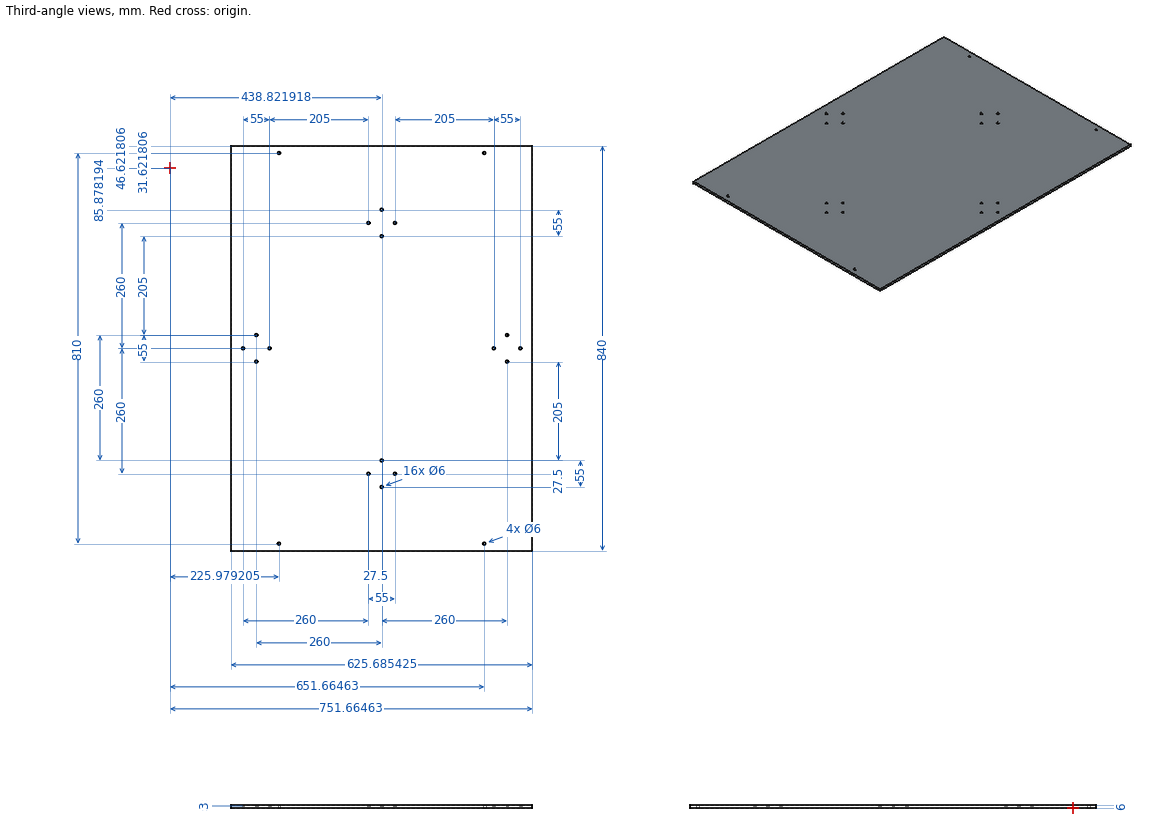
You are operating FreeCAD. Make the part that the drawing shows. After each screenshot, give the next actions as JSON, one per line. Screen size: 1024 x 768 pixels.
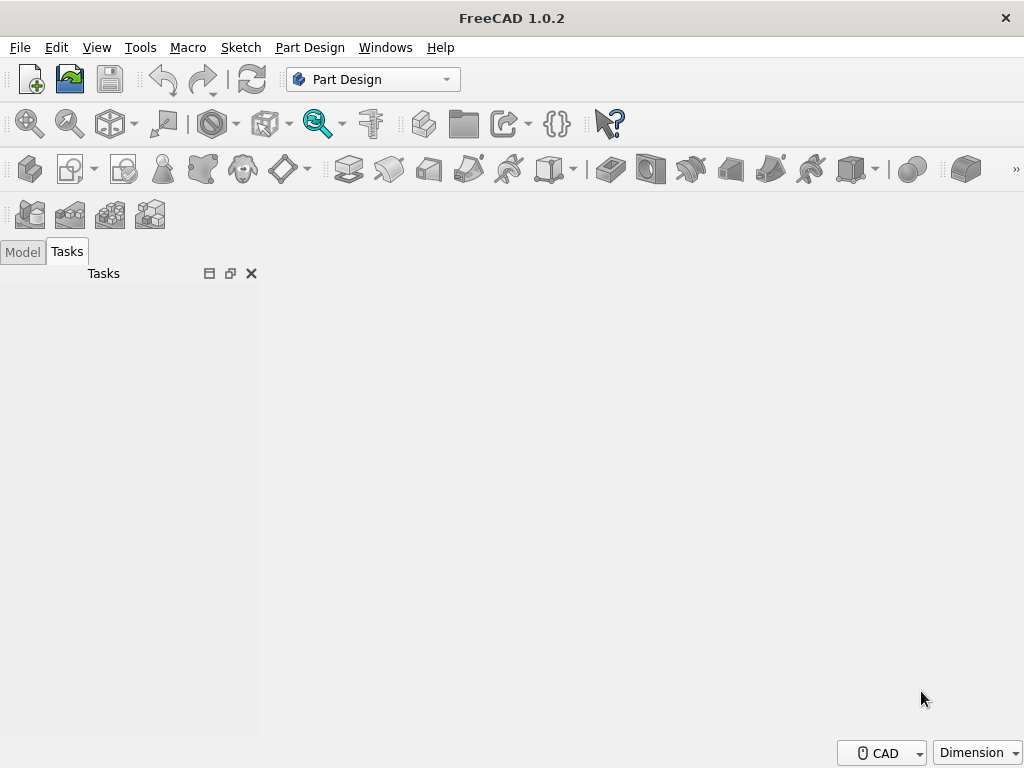
{"action": "left_click", "coordinate": [30, 80]}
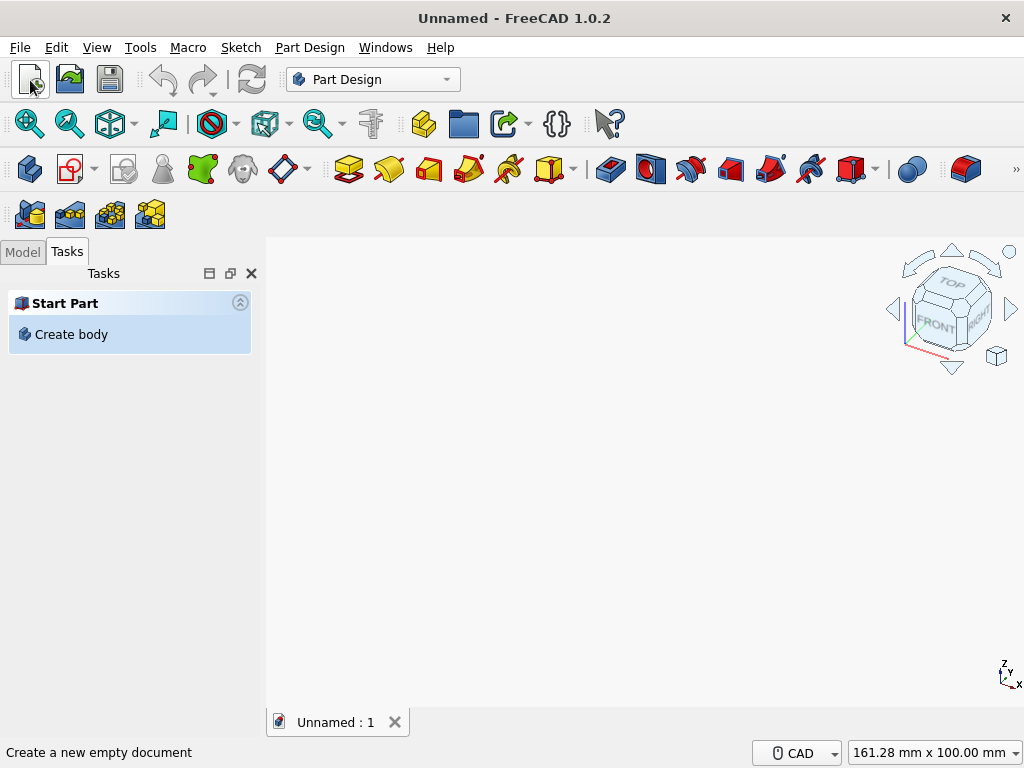
{"action": "left_click", "coordinate": [70, 170]}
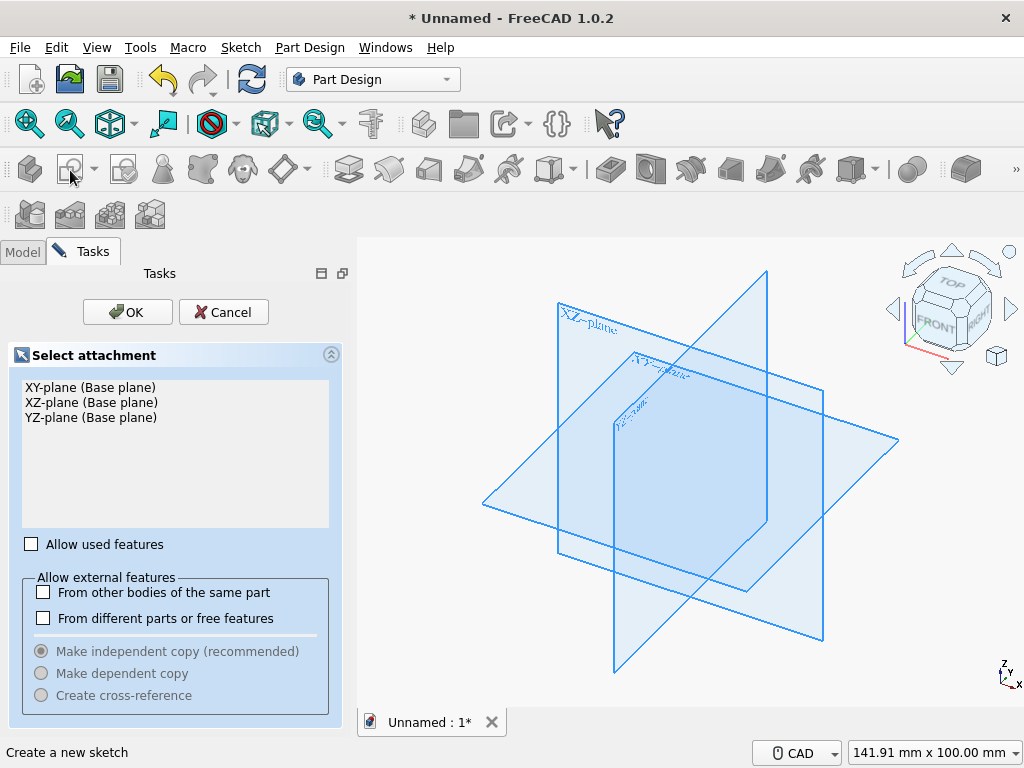
{"action": "left_click", "coordinate": [82, 388]}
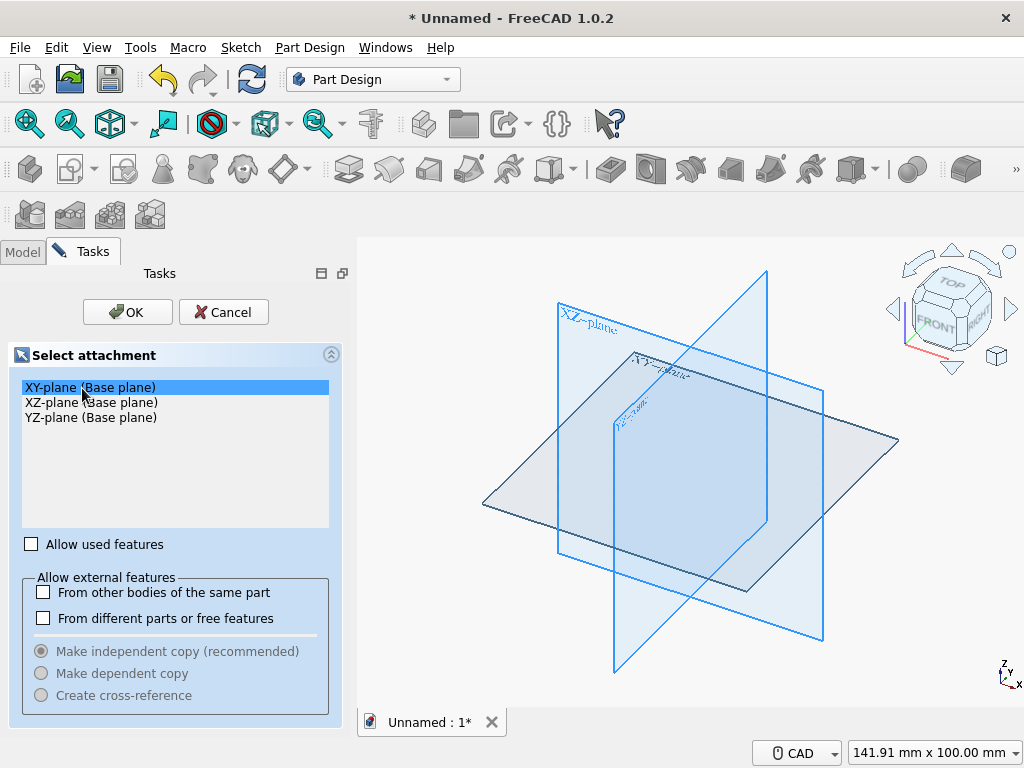
{"action": "left_click", "coordinate": [128, 312]}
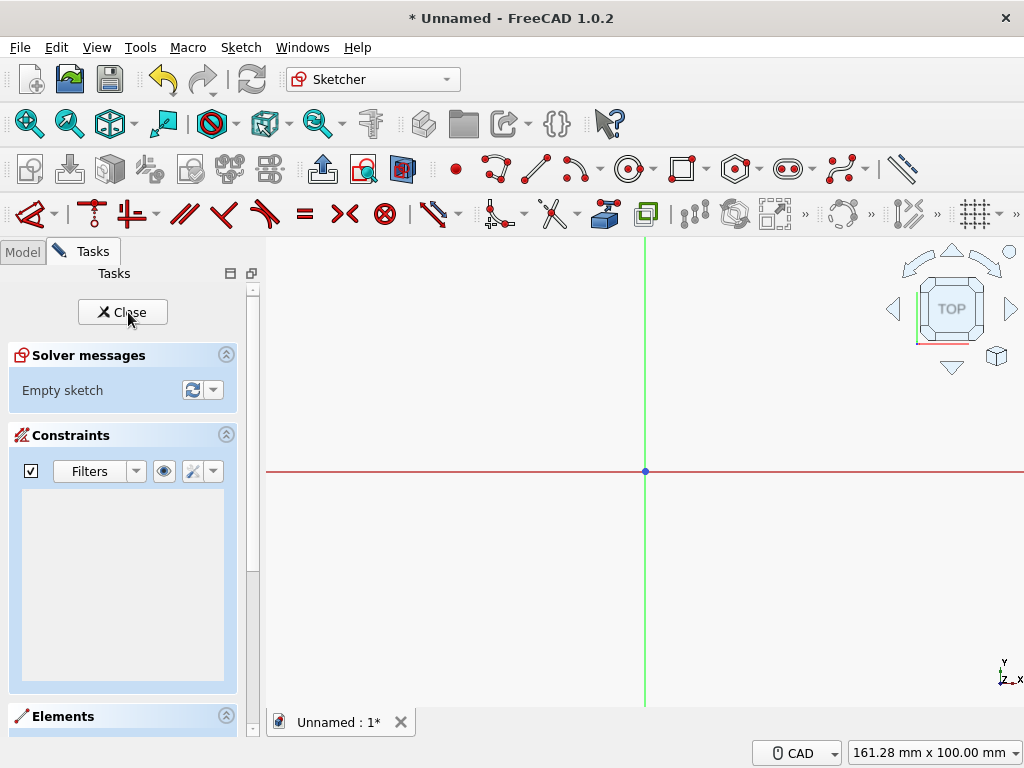
{"action": "scroll", "coordinate": [429, 331], "scroll_direction": "down", "scroll_amount": 13}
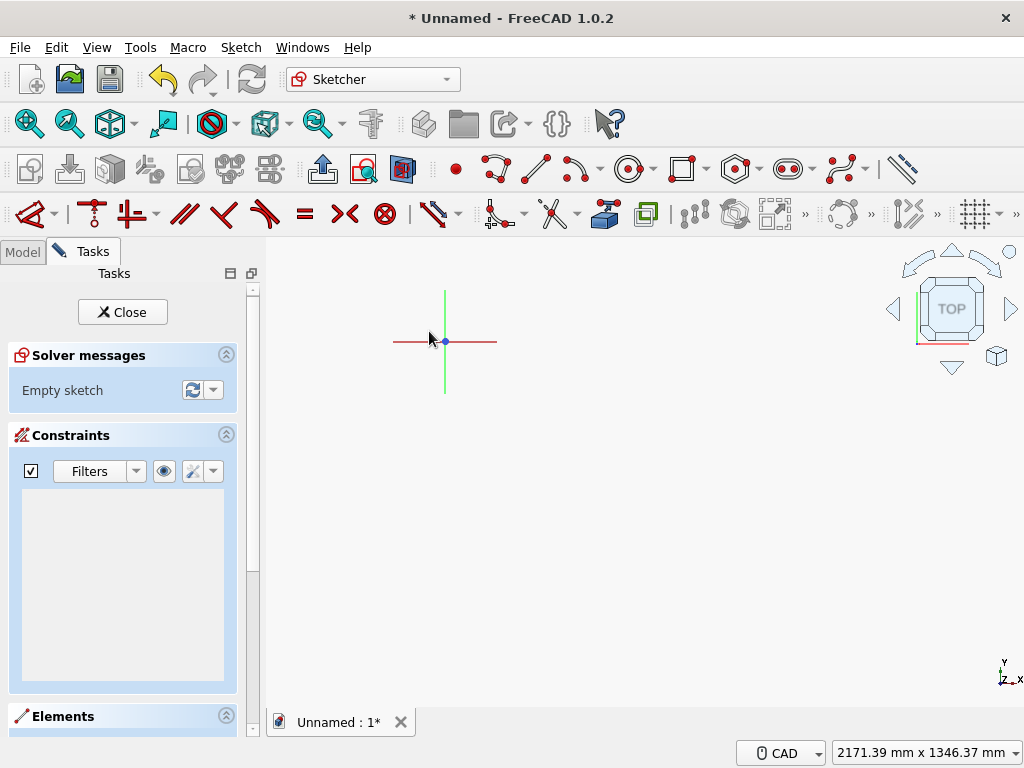
{"action": "left_click", "coordinate": [682, 170]}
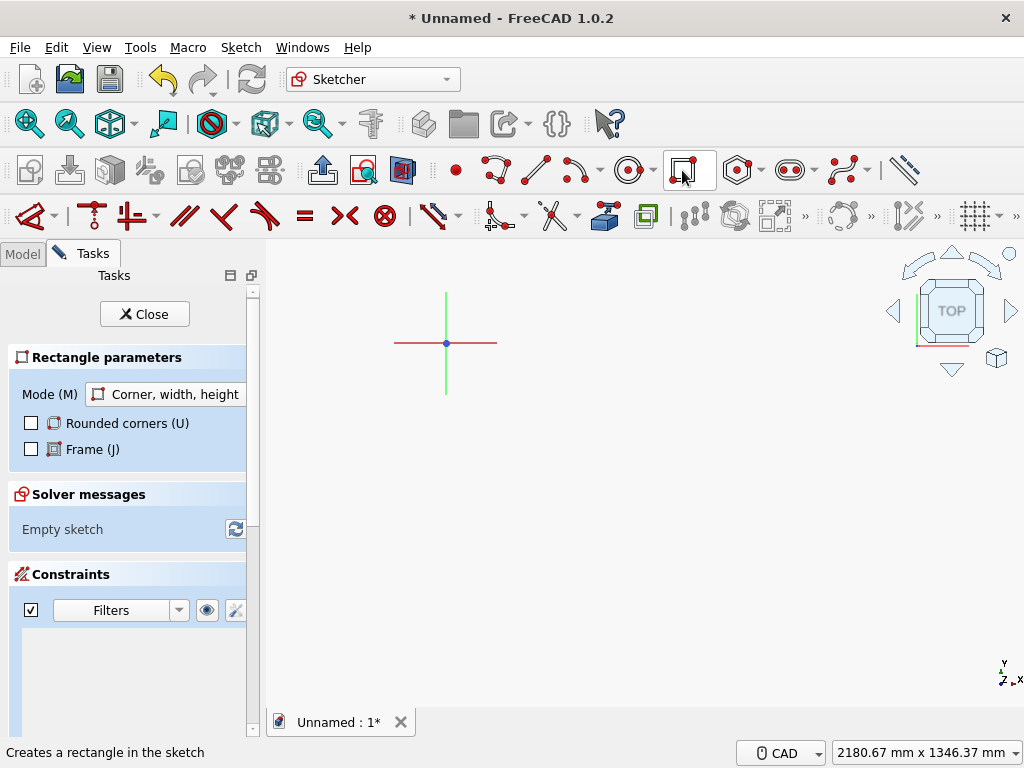
{"action": "left_click", "coordinate": [490, 327]}
{"action": "mouse_move", "coordinate": [707, 619]}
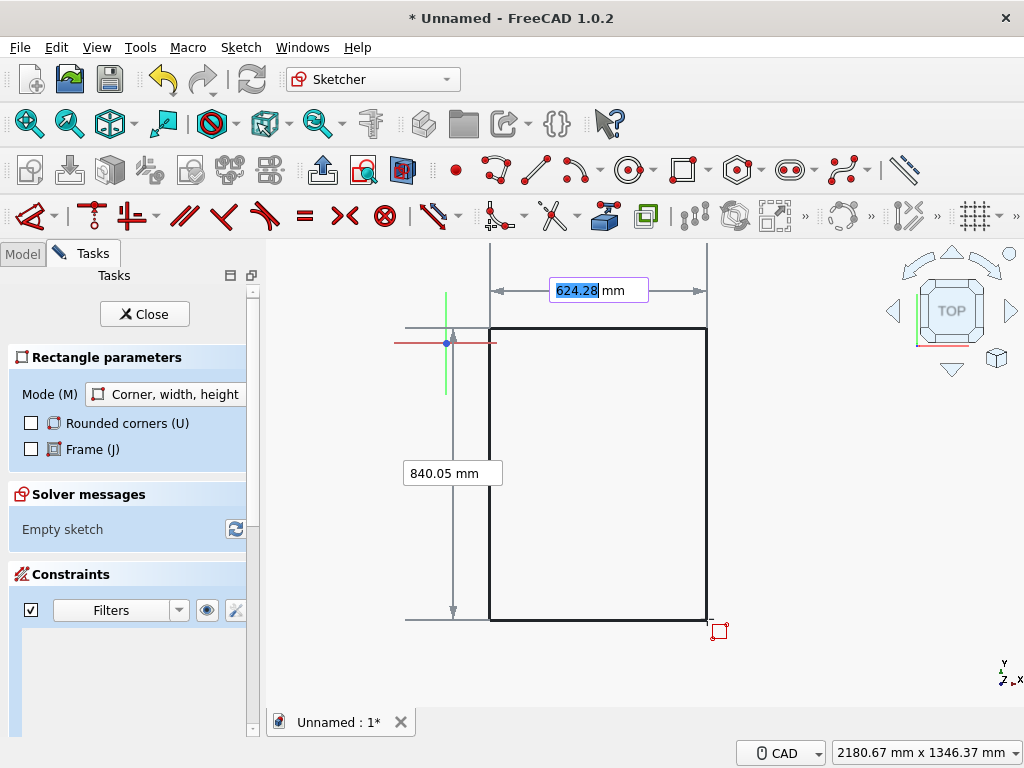
{"action": "type", "text": "625.685425"}
{"action": "key", "text": "Tab"}
{"action": "type", "text": "840"}
{"action": "key", "text": "Return"}
{"action": "key", "text": "Escape"}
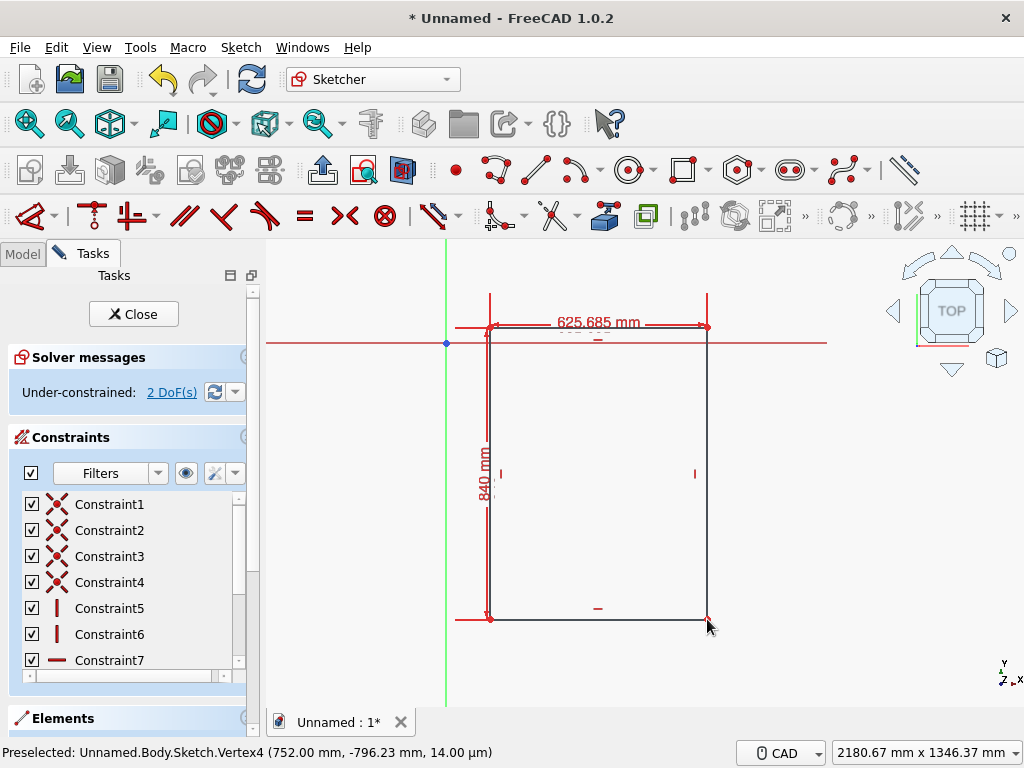
{"action": "left_click", "coordinate": [30, 216]}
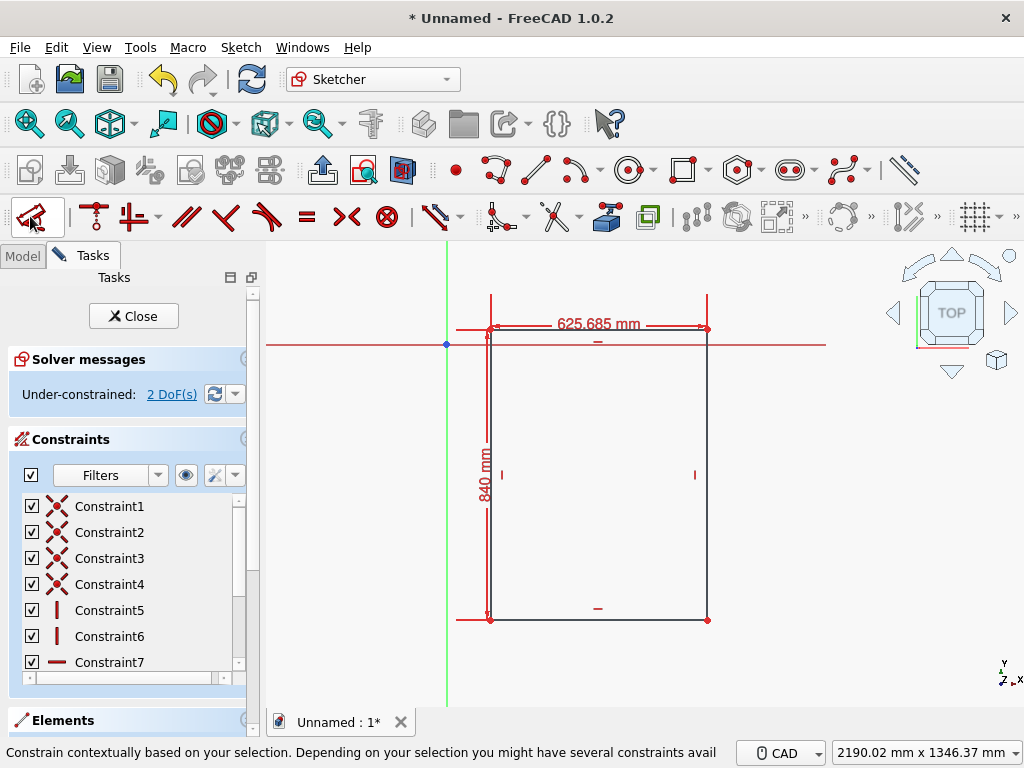
{"action": "scroll", "coordinate": [491, 330], "scroll_direction": "up", "scroll_amount": 5}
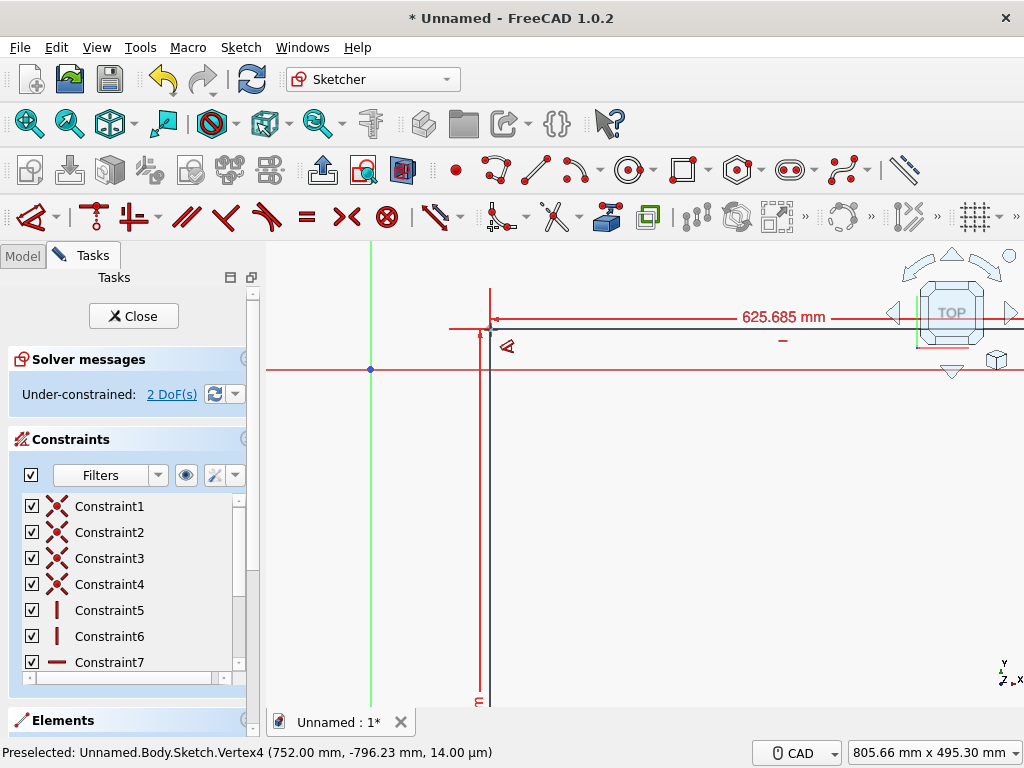
{"action": "left_click", "coordinate": [490, 329]}
{"action": "left_click", "coordinate": [337, 349]}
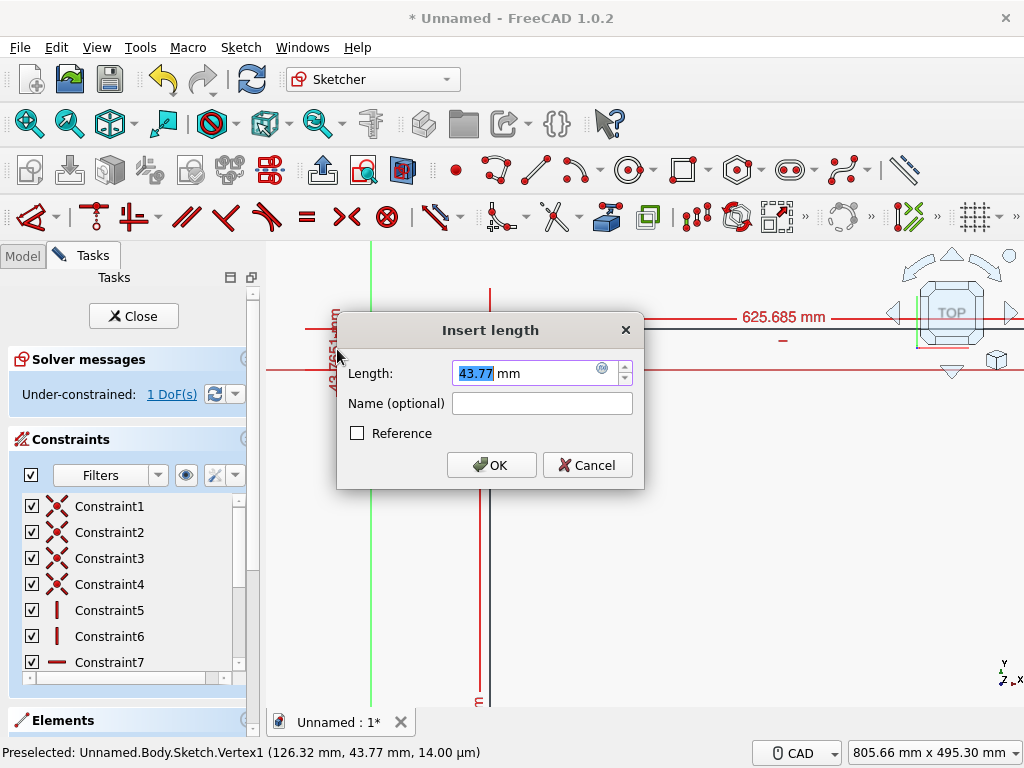
{"action": "type", "text": "46.621806"}
{"action": "key", "text": "Return"}